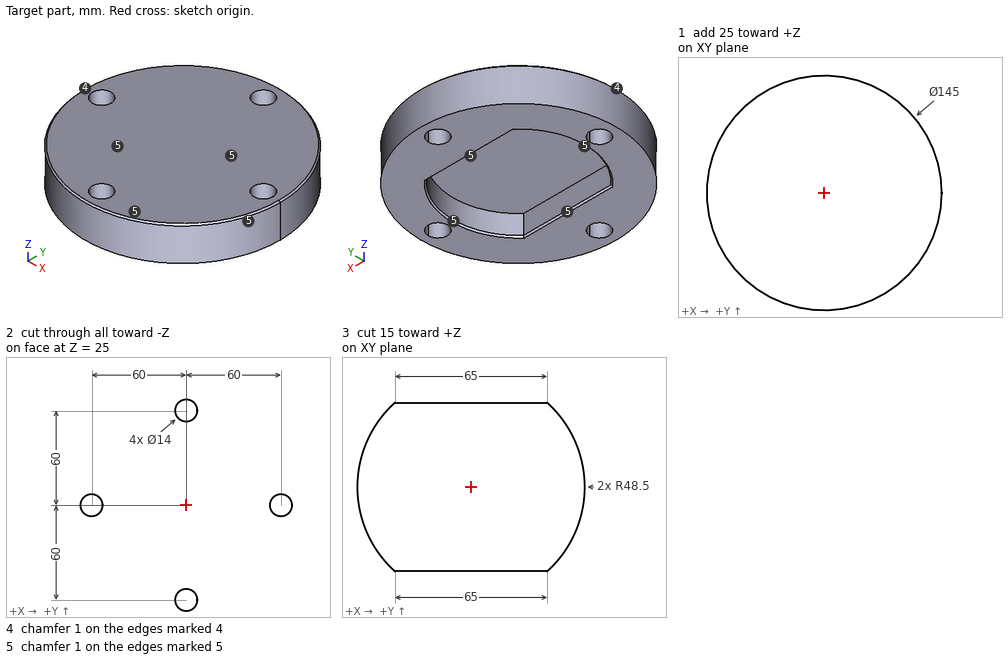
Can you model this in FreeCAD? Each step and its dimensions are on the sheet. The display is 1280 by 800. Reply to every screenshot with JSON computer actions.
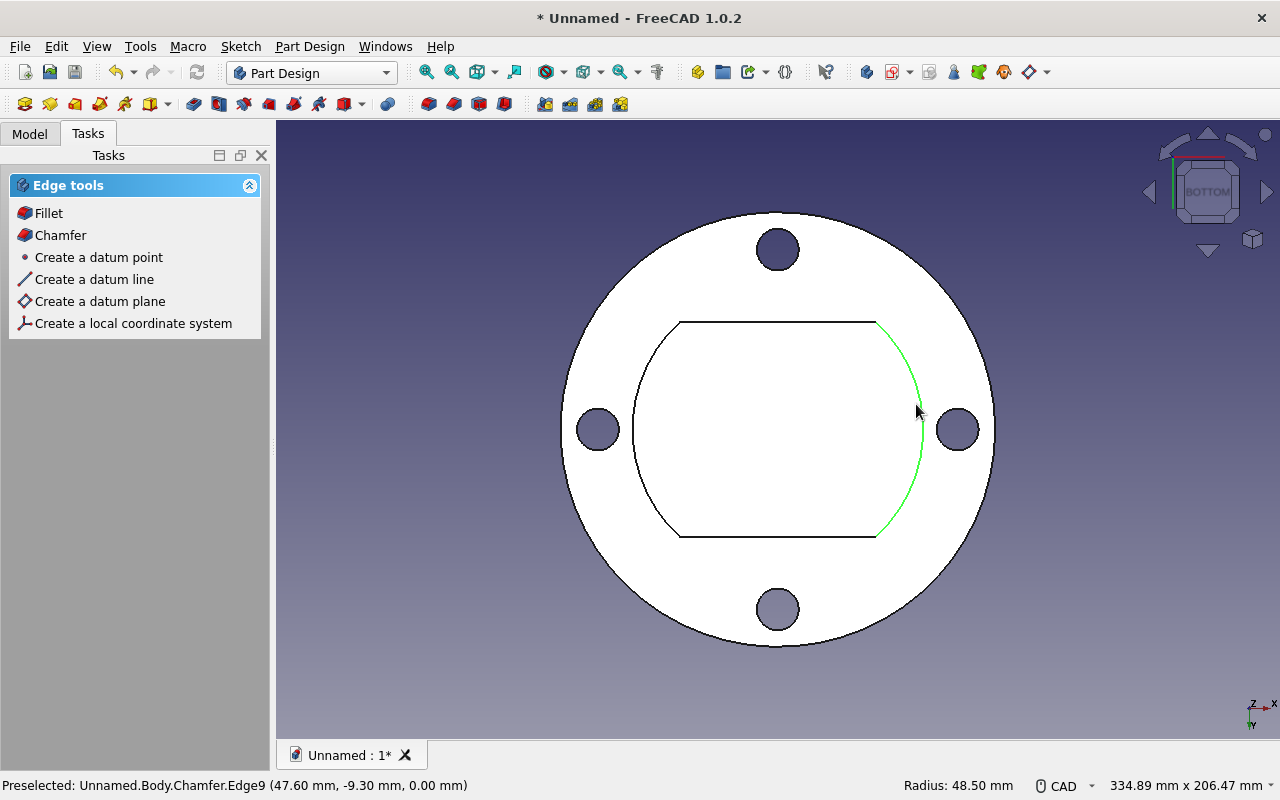
{"action": "left_click", "coordinate": [778, 321], "text": "ctrl"}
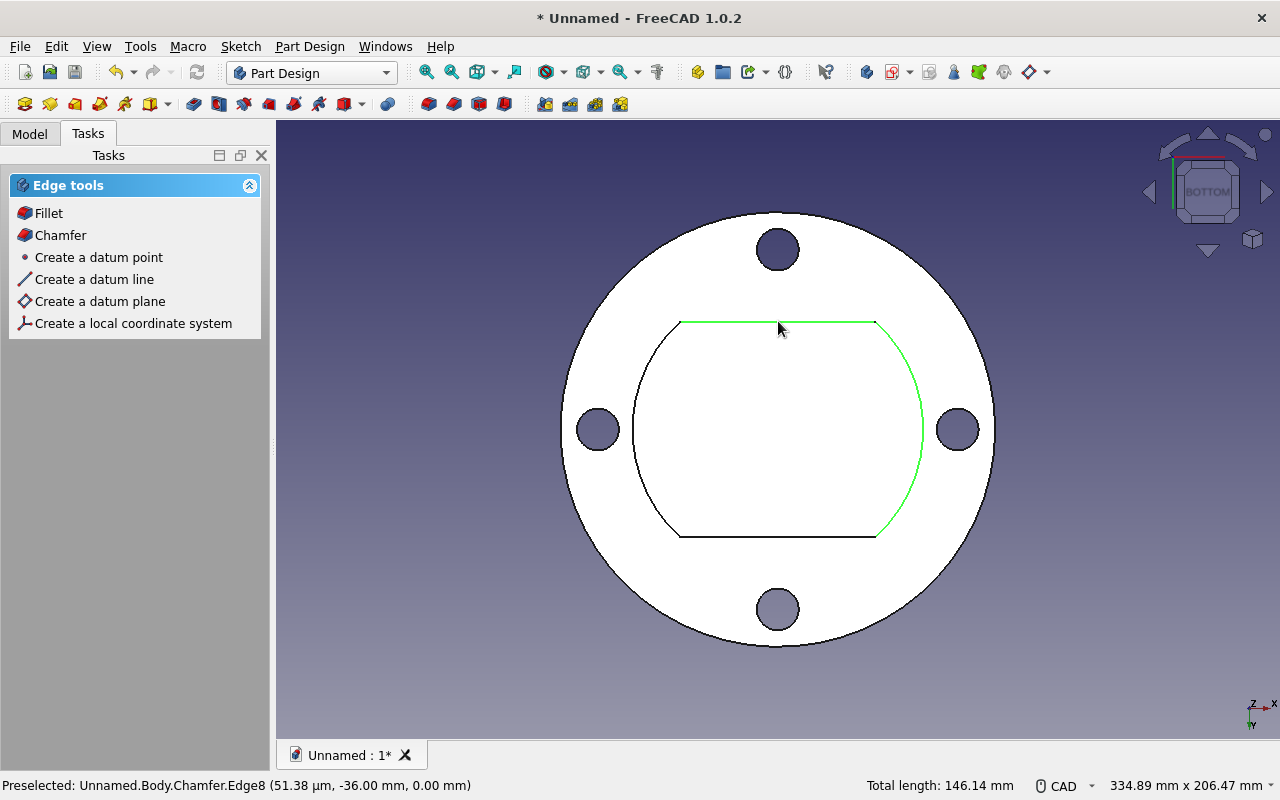
{"action": "left_click", "coordinate": [634, 453], "text": "ctrl"}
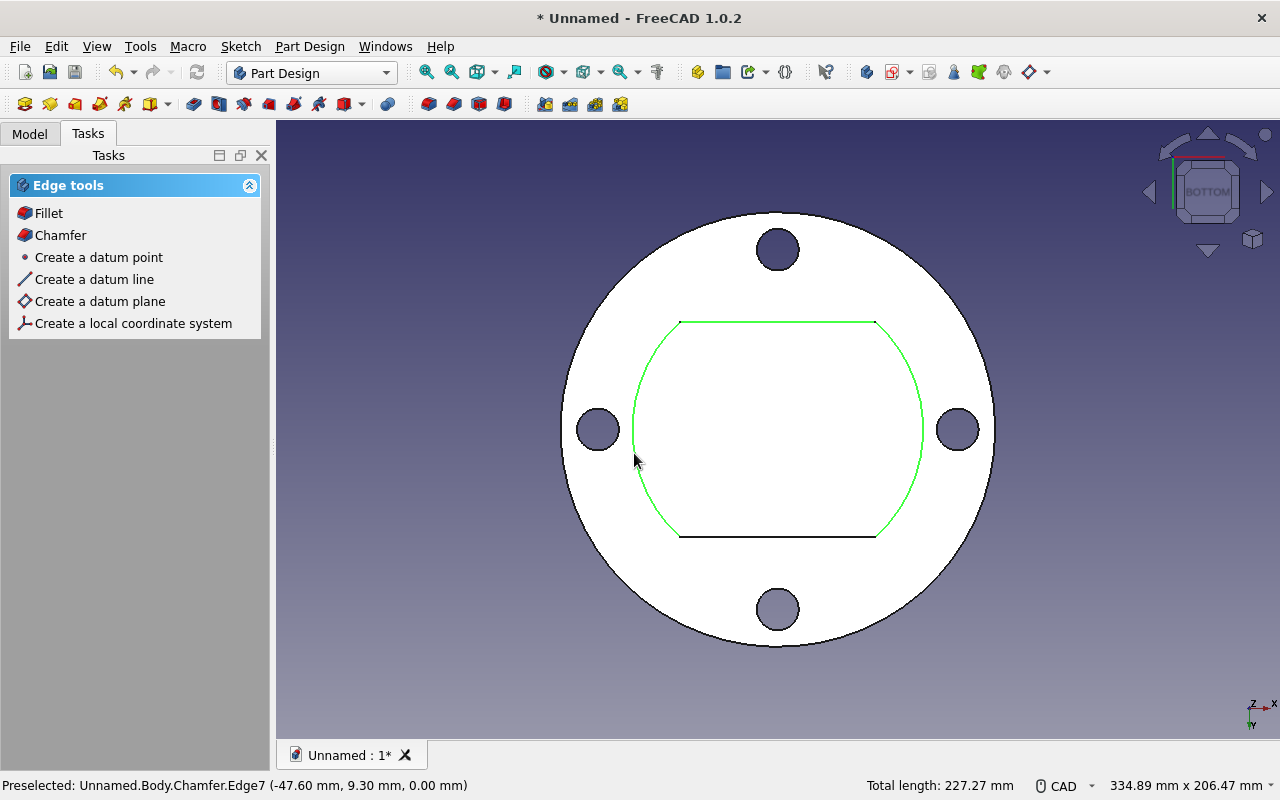
{"action": "left_click", "coordinate": [778, 536], "text": "ctrl"}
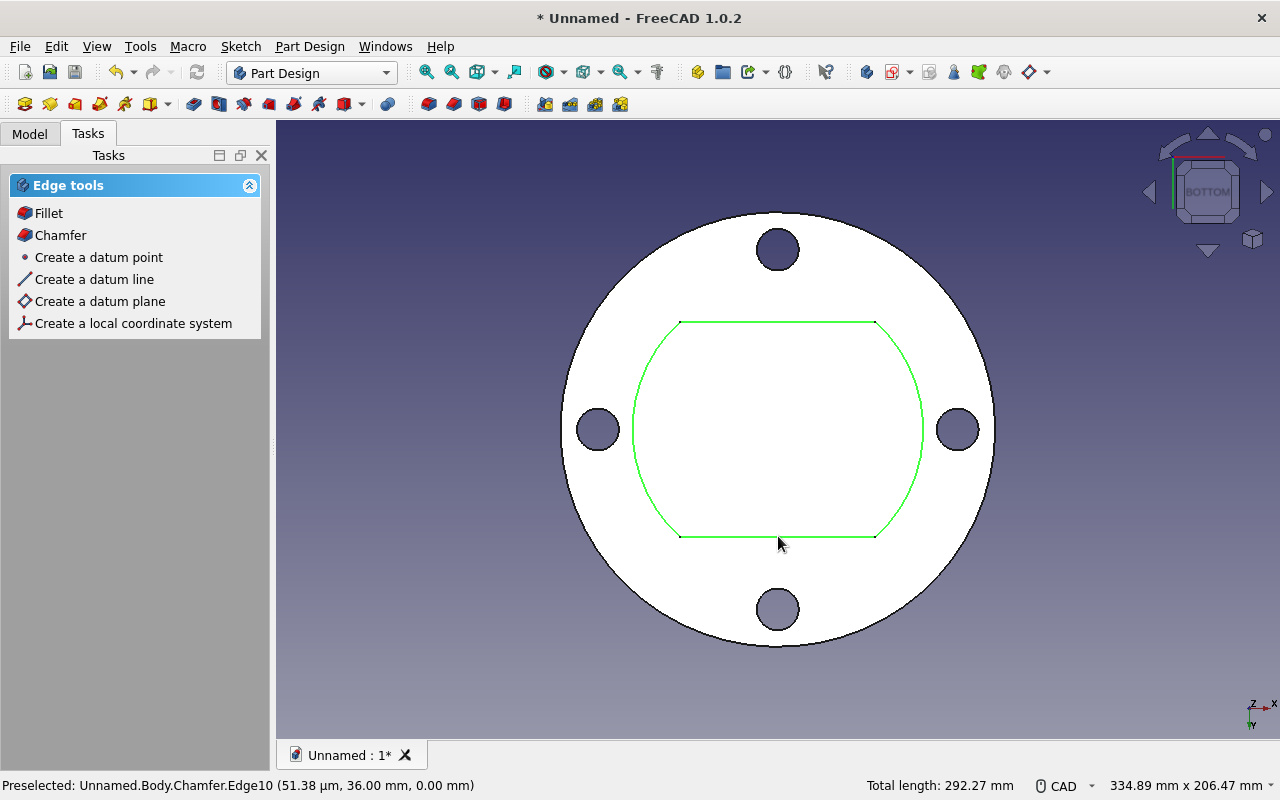
{"action": "left_click", "coordinate": [454, 104]}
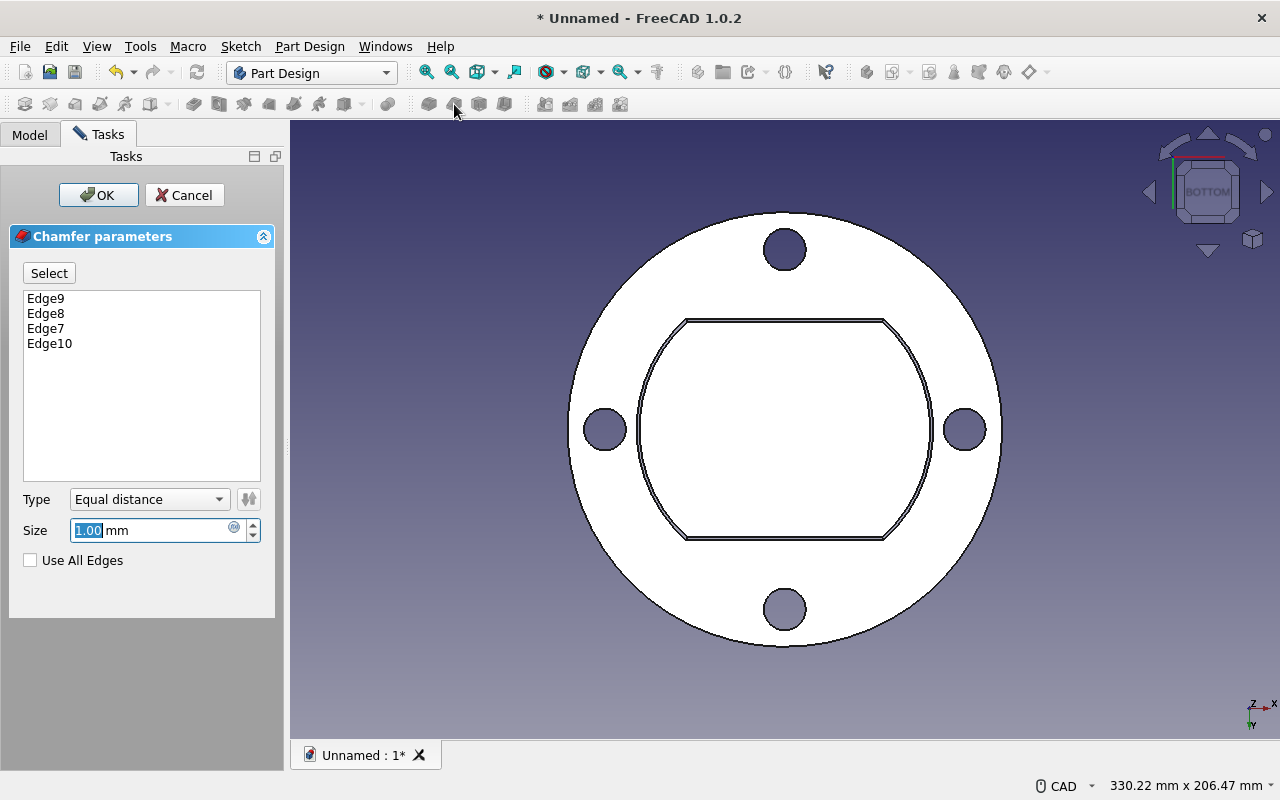
{"action": "type", "text": "1"}
{"action": "key", "text": "Tab"}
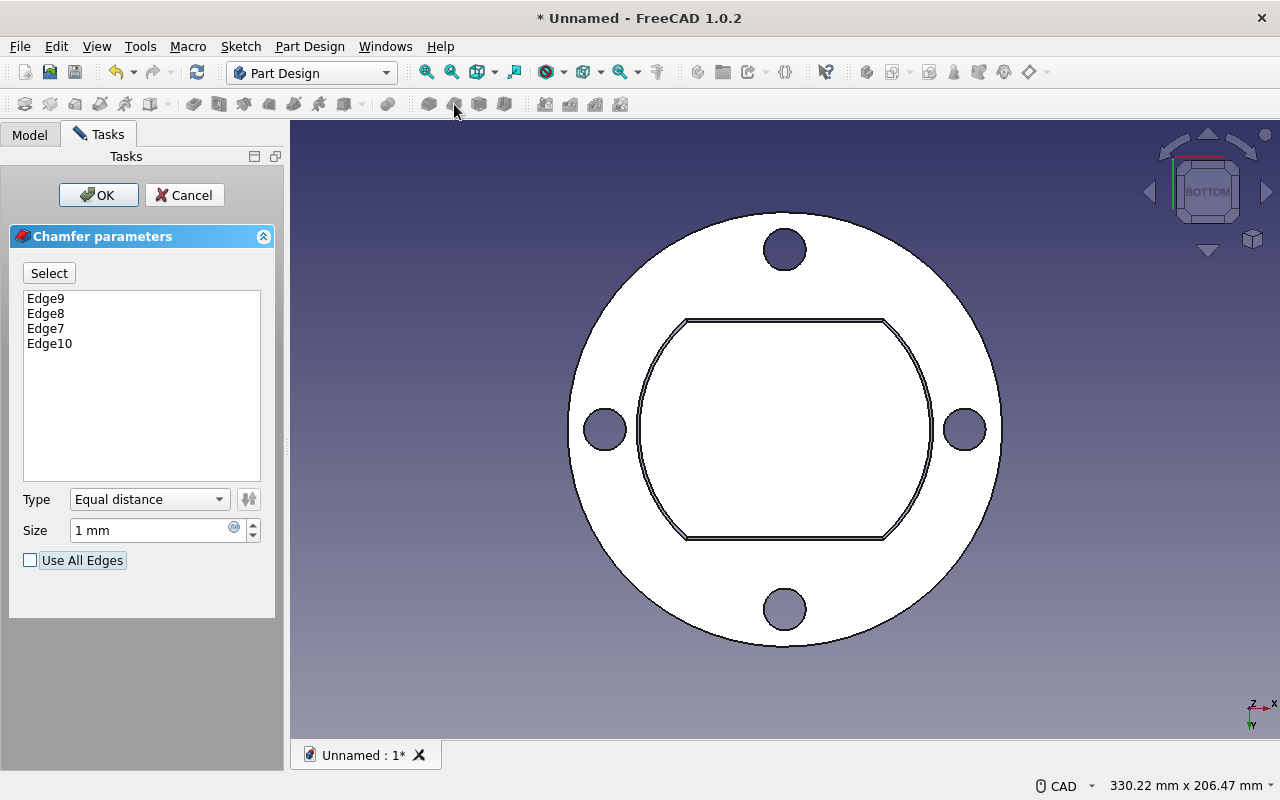
{"action": "left_click", "coordinate": [99, 195]}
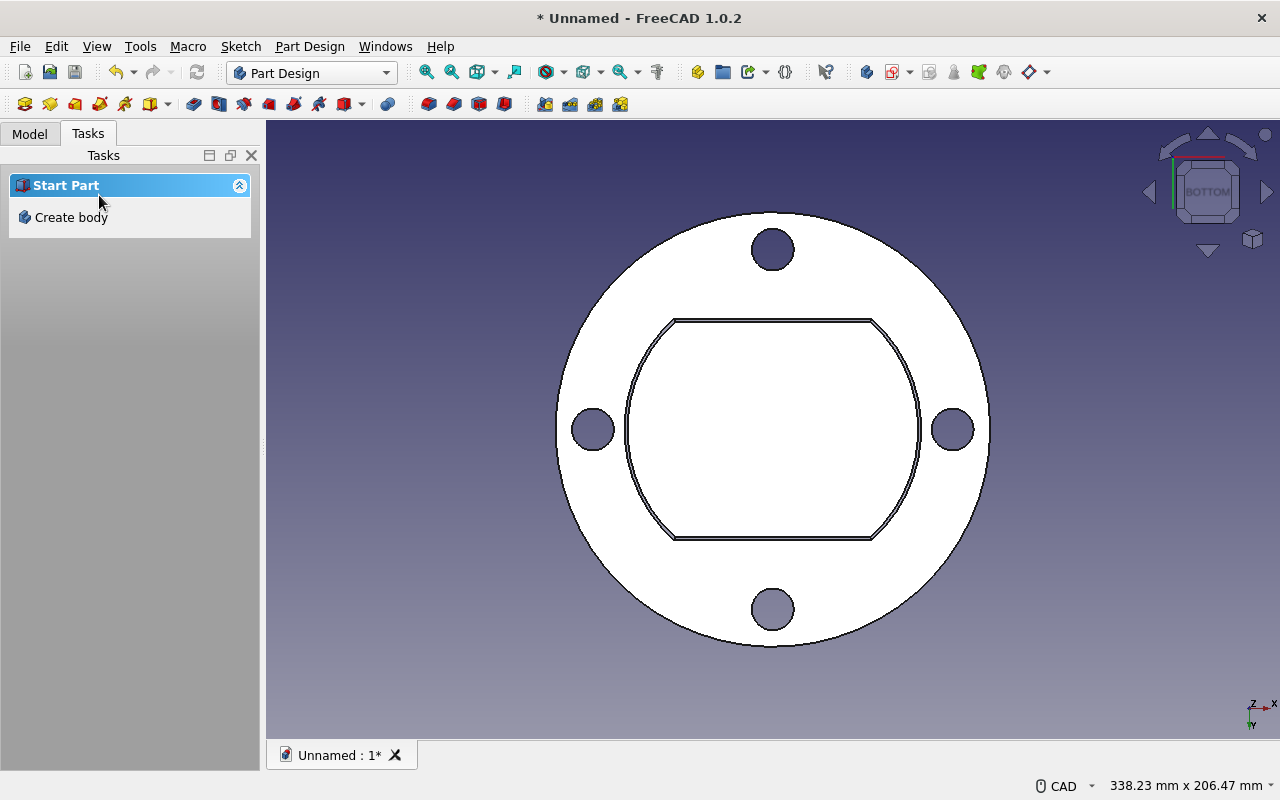
{"action": "key", "text": "0"}